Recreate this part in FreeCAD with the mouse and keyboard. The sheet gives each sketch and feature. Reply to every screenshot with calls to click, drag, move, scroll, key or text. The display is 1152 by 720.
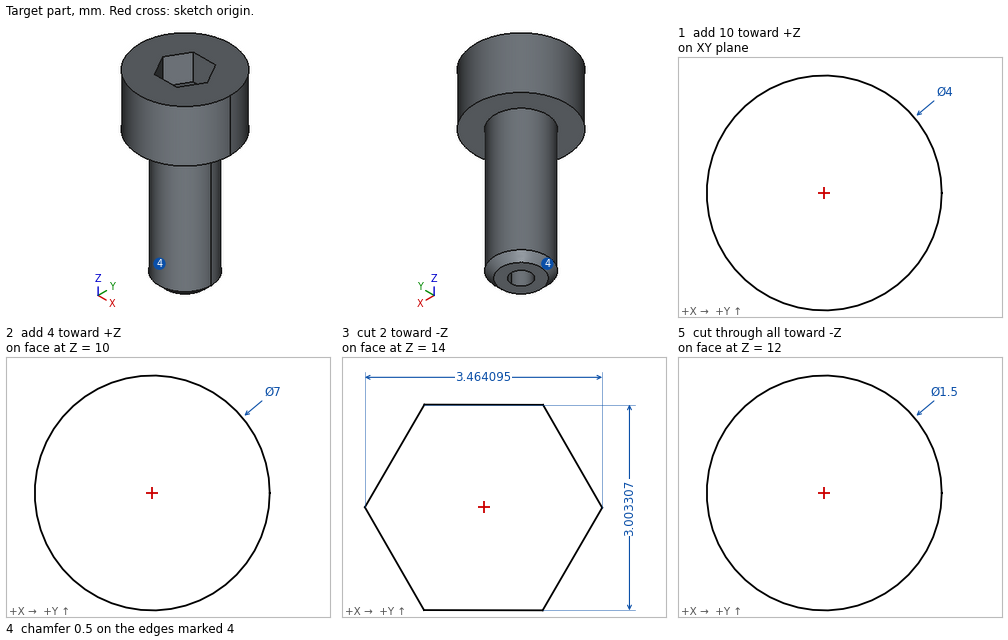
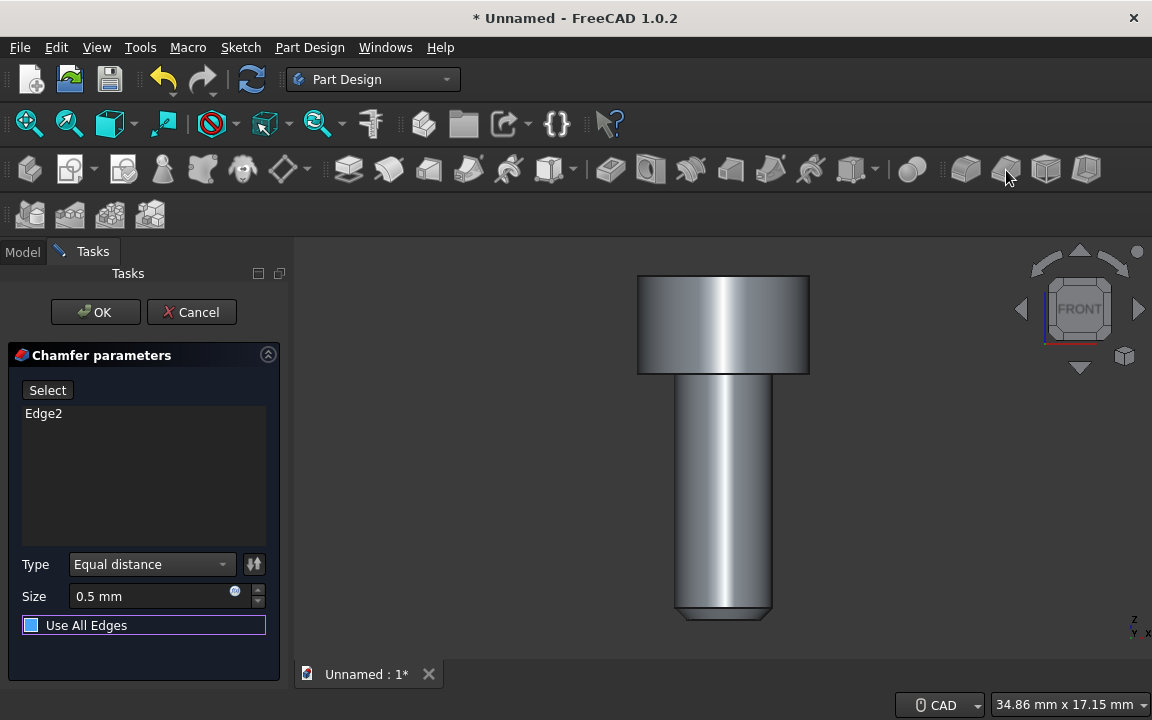
click(96, 312)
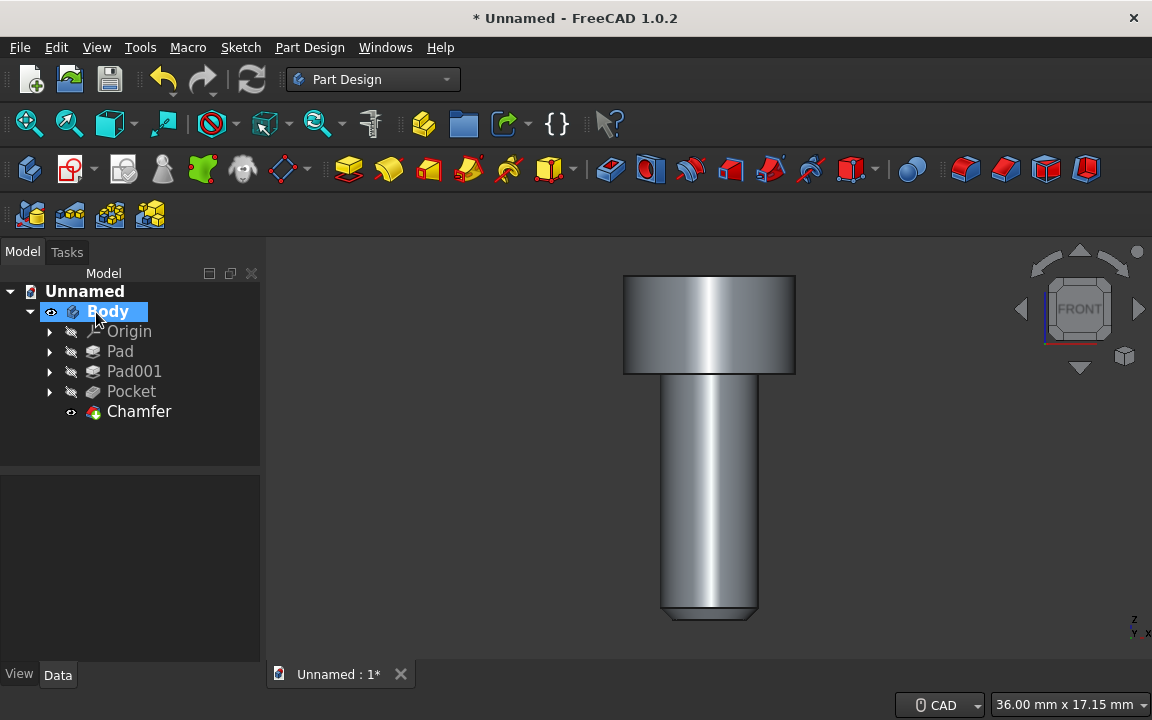
key(0)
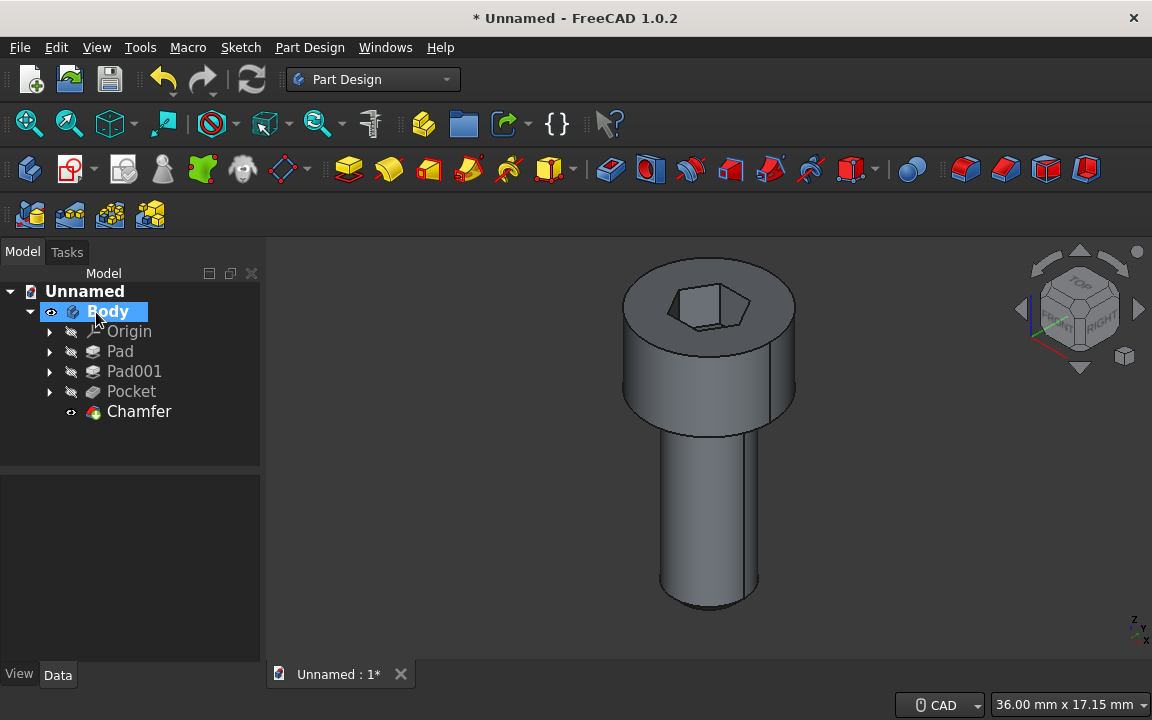
click(30, 124)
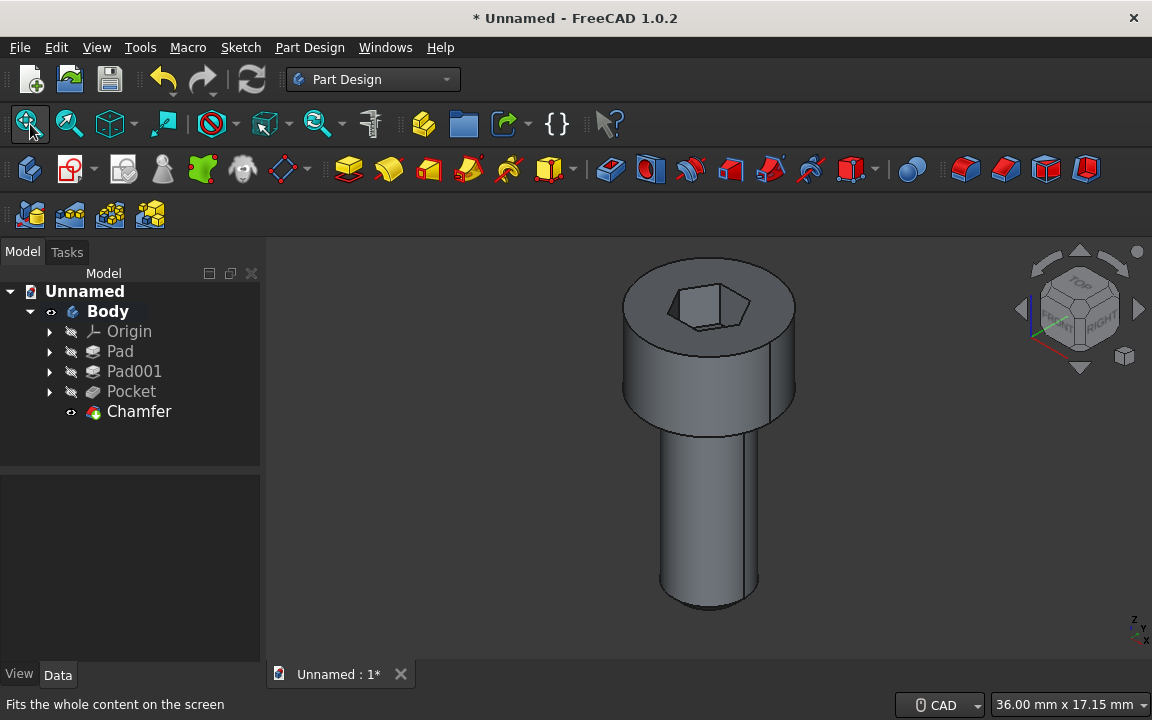
key(2)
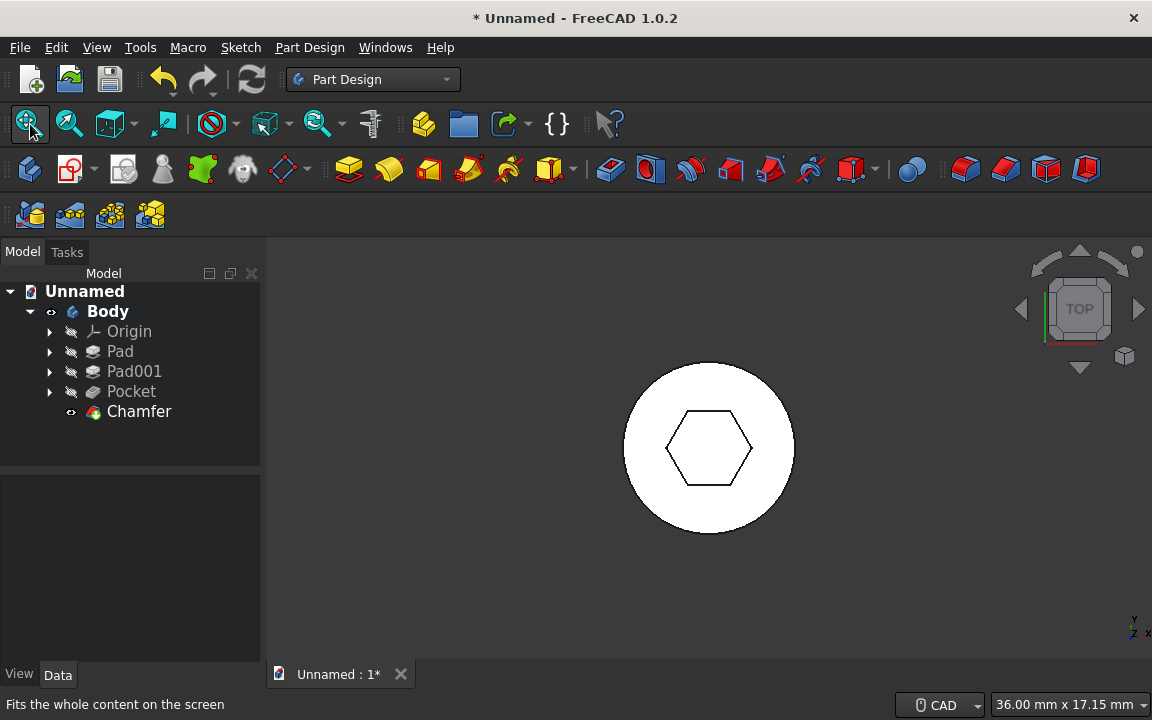
click(30, 124)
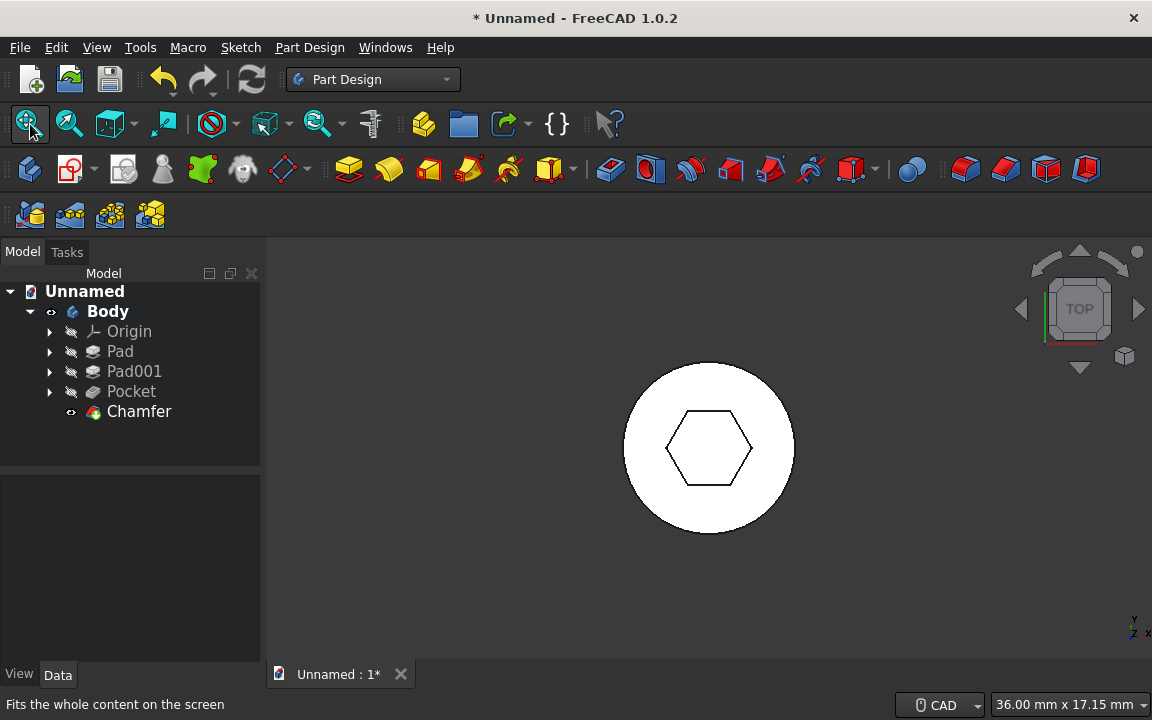
click(709, 447)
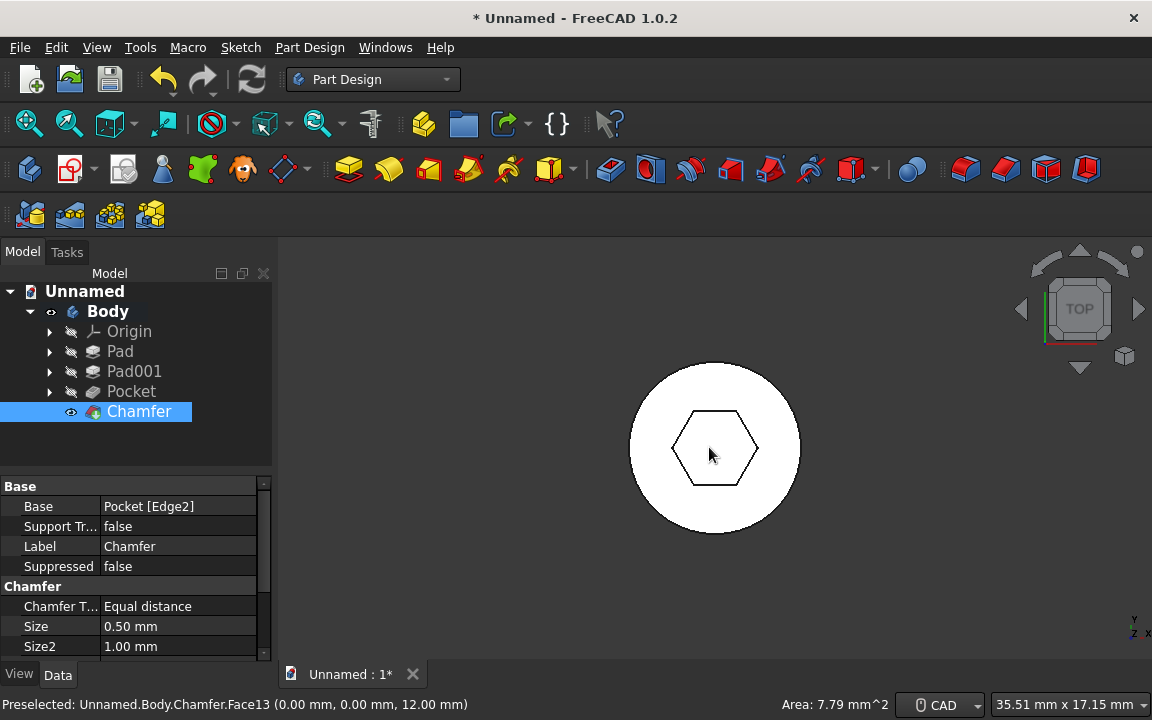
click(70, 170)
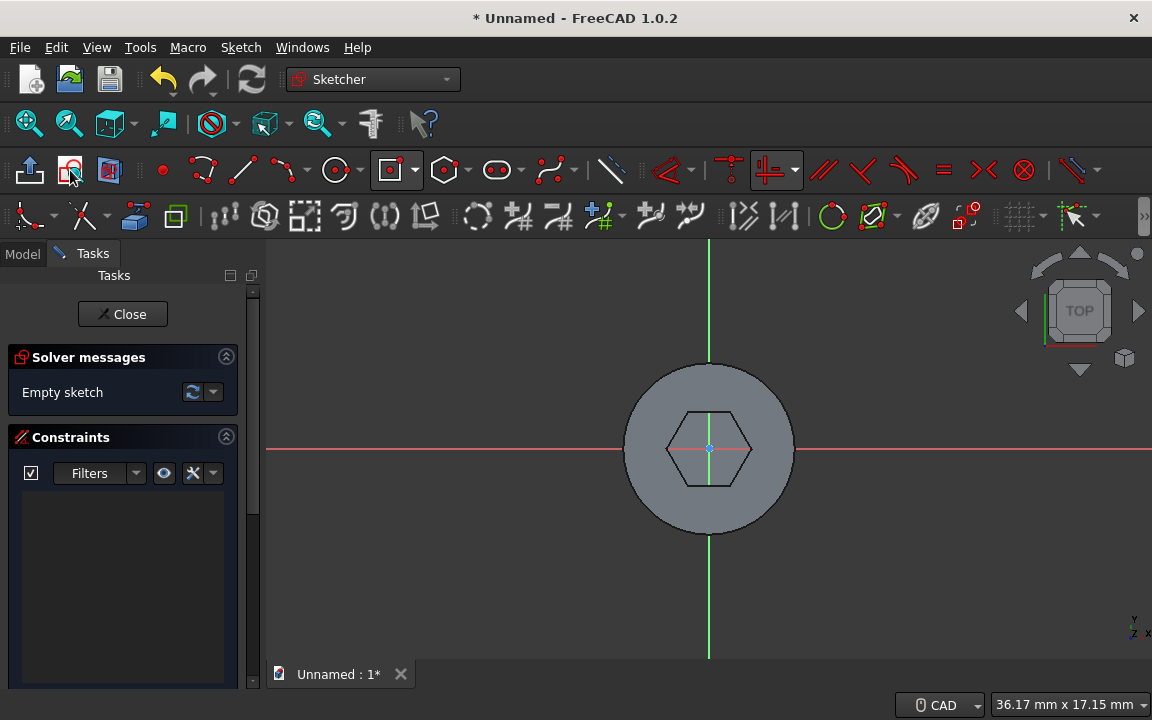
click(110, 170)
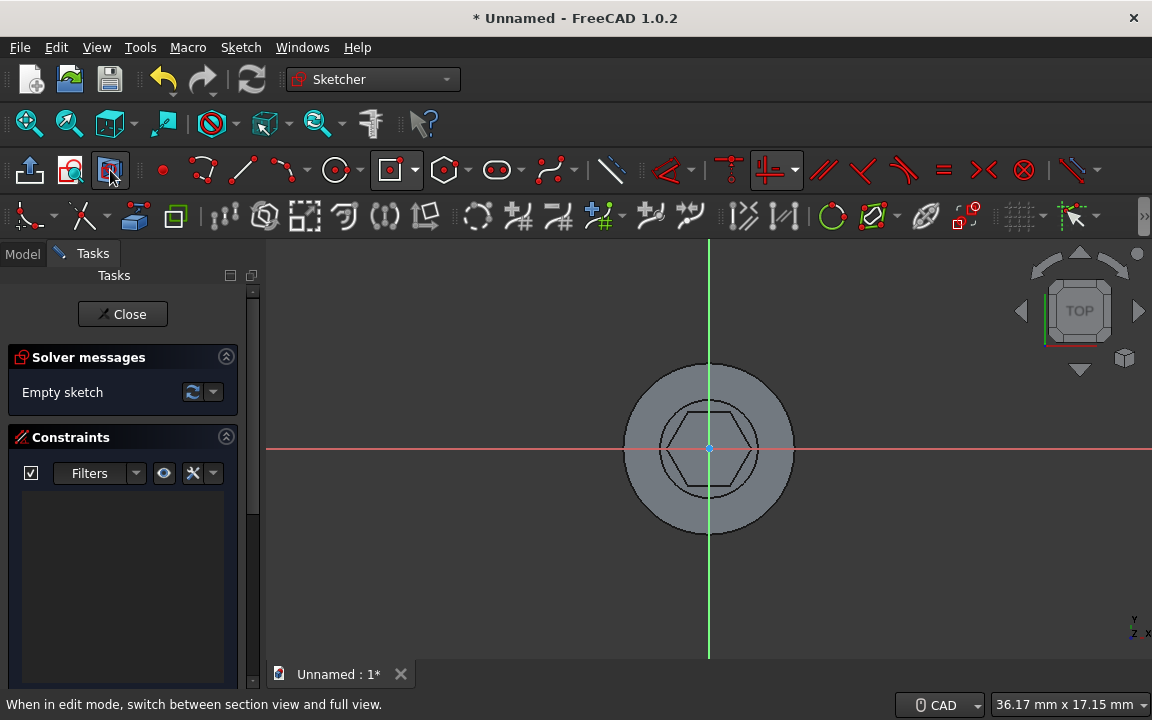
scroll(720, 449, up, 10)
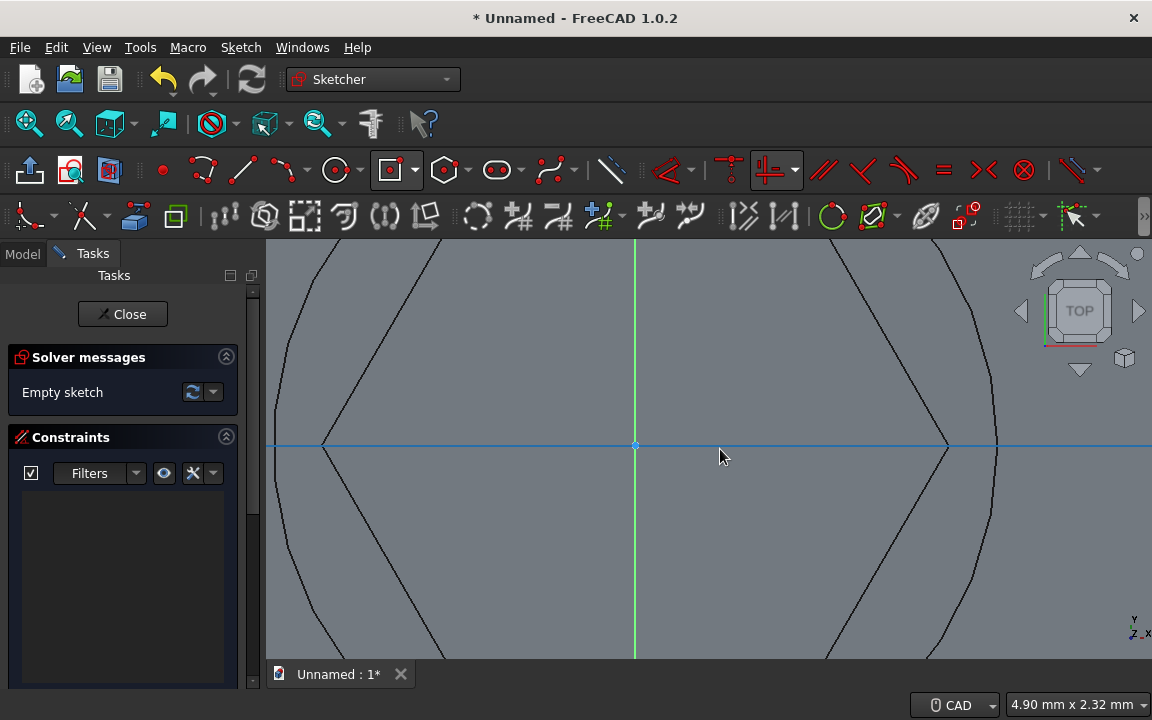
click(336, 170)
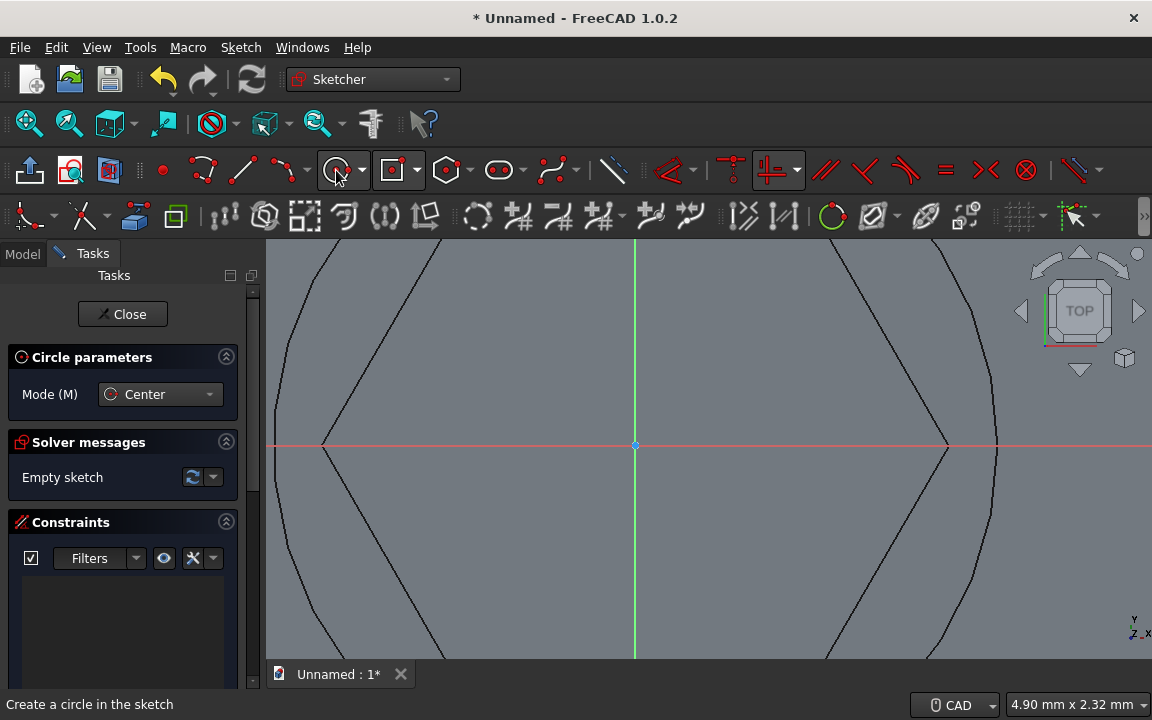
click(635, 446)
move(731, 350)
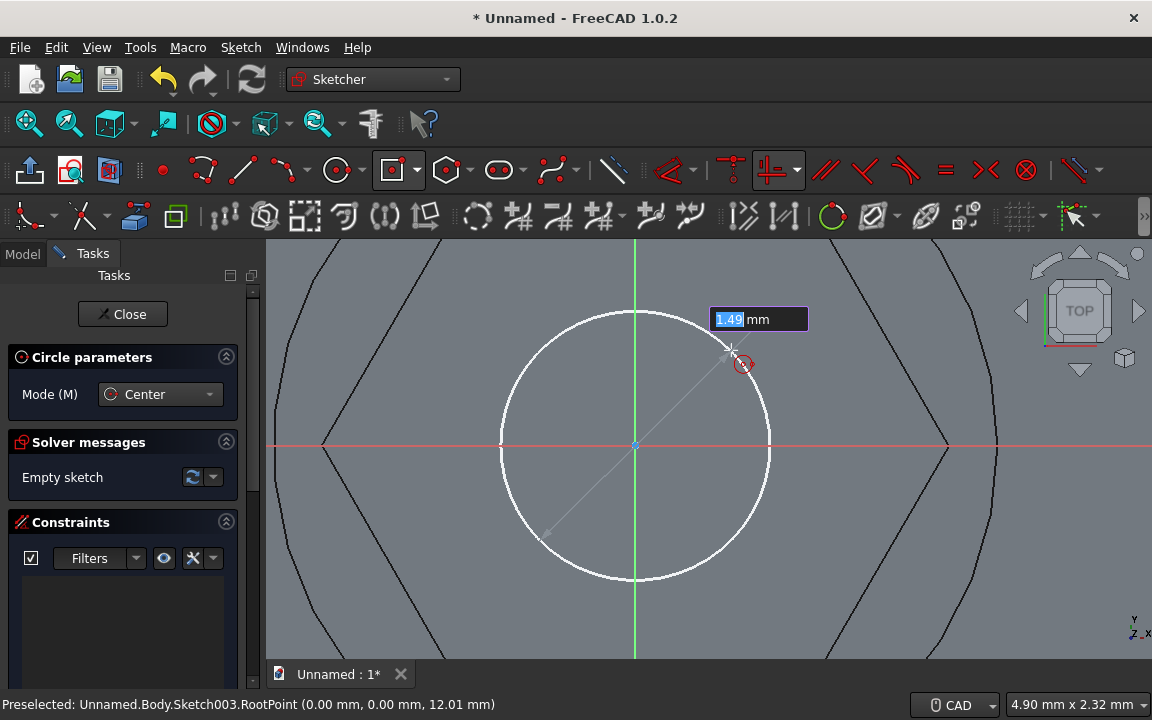
text(1.5)
key(Return)
key(Escape)